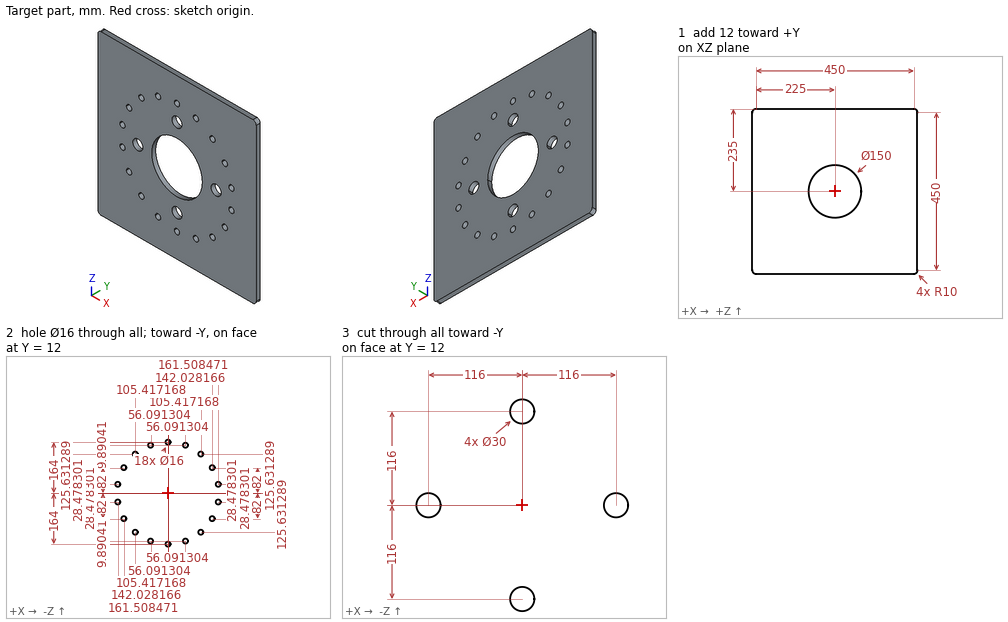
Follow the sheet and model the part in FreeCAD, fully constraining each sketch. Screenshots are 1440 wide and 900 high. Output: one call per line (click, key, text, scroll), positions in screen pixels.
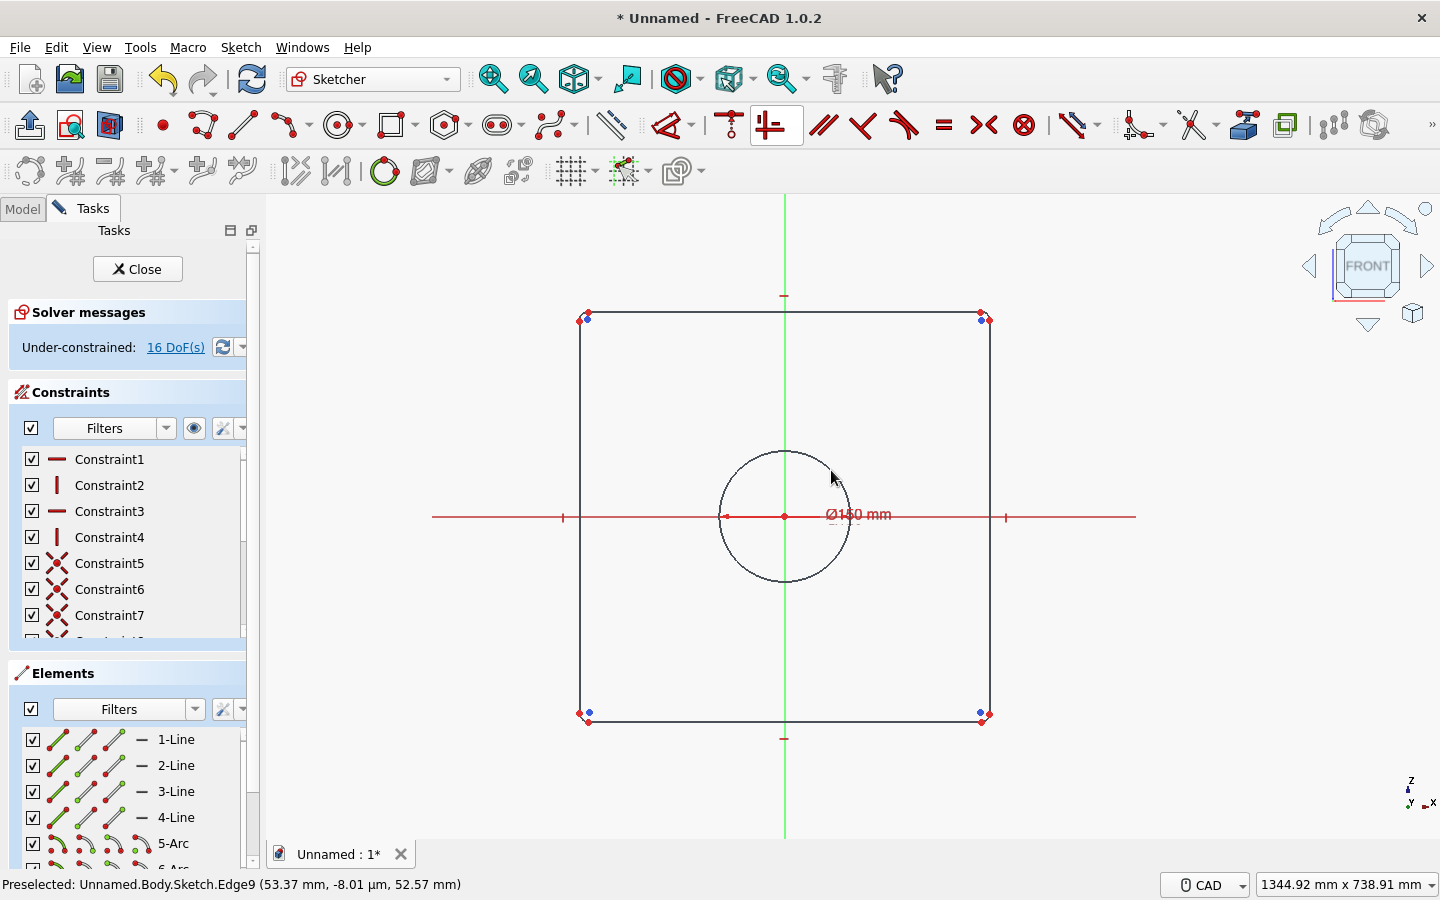
click(706, 312)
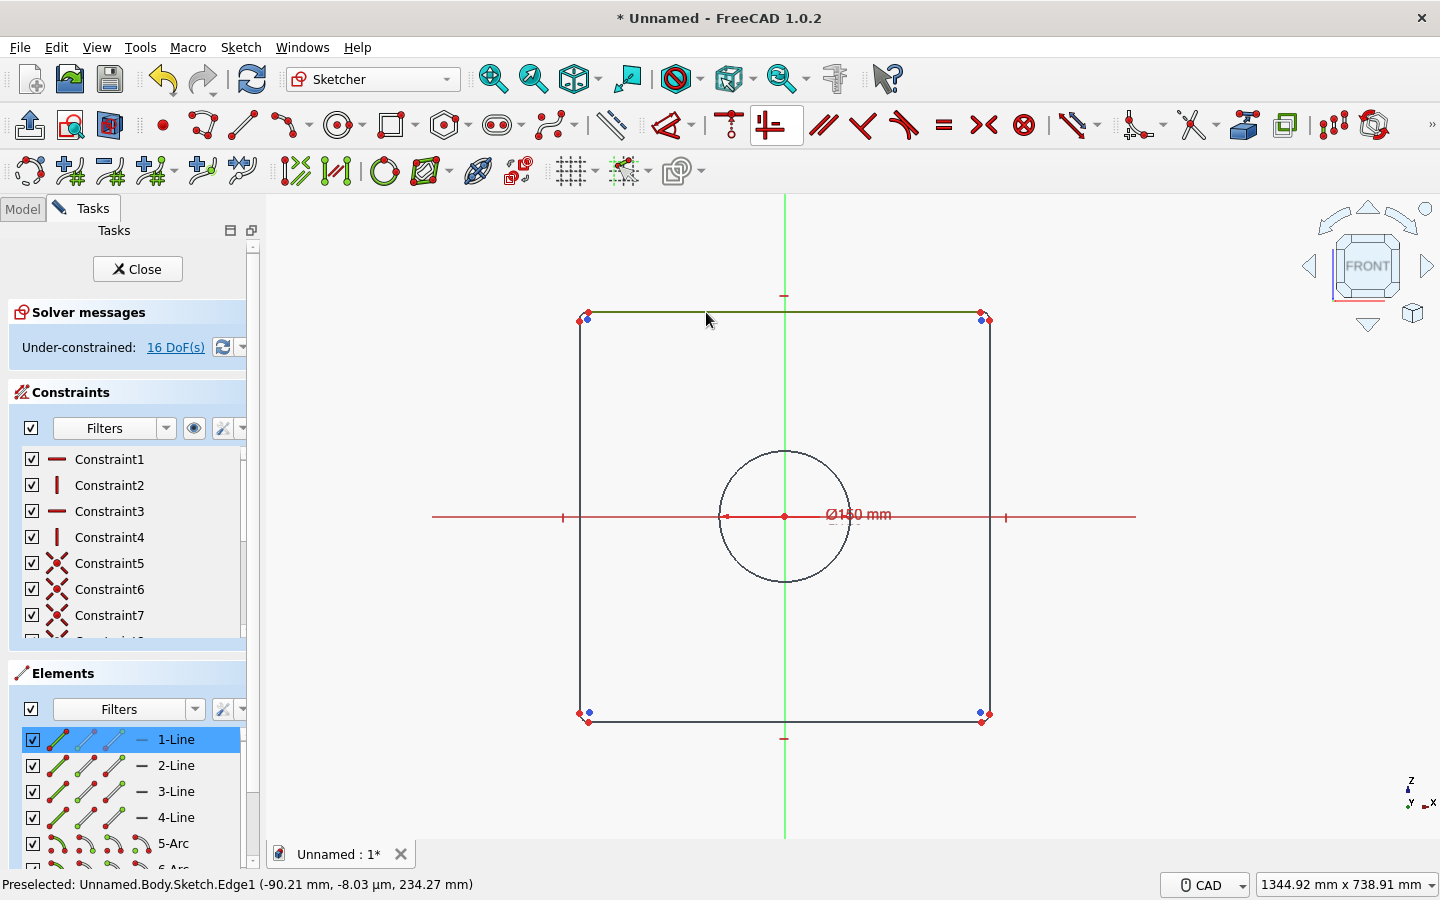
scroll(987, 314, up, 4)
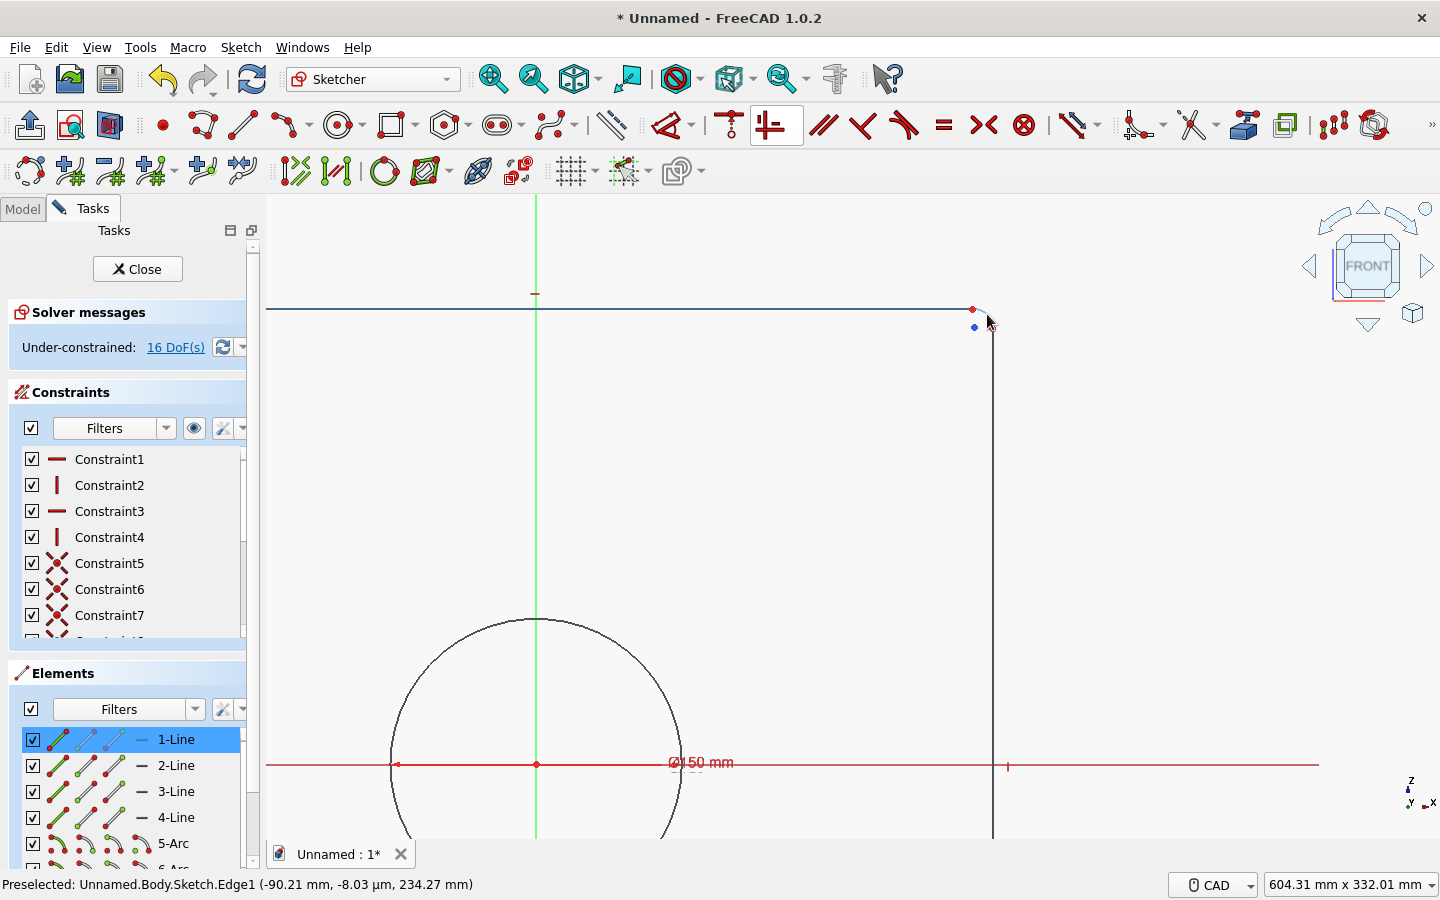
click(987, 314)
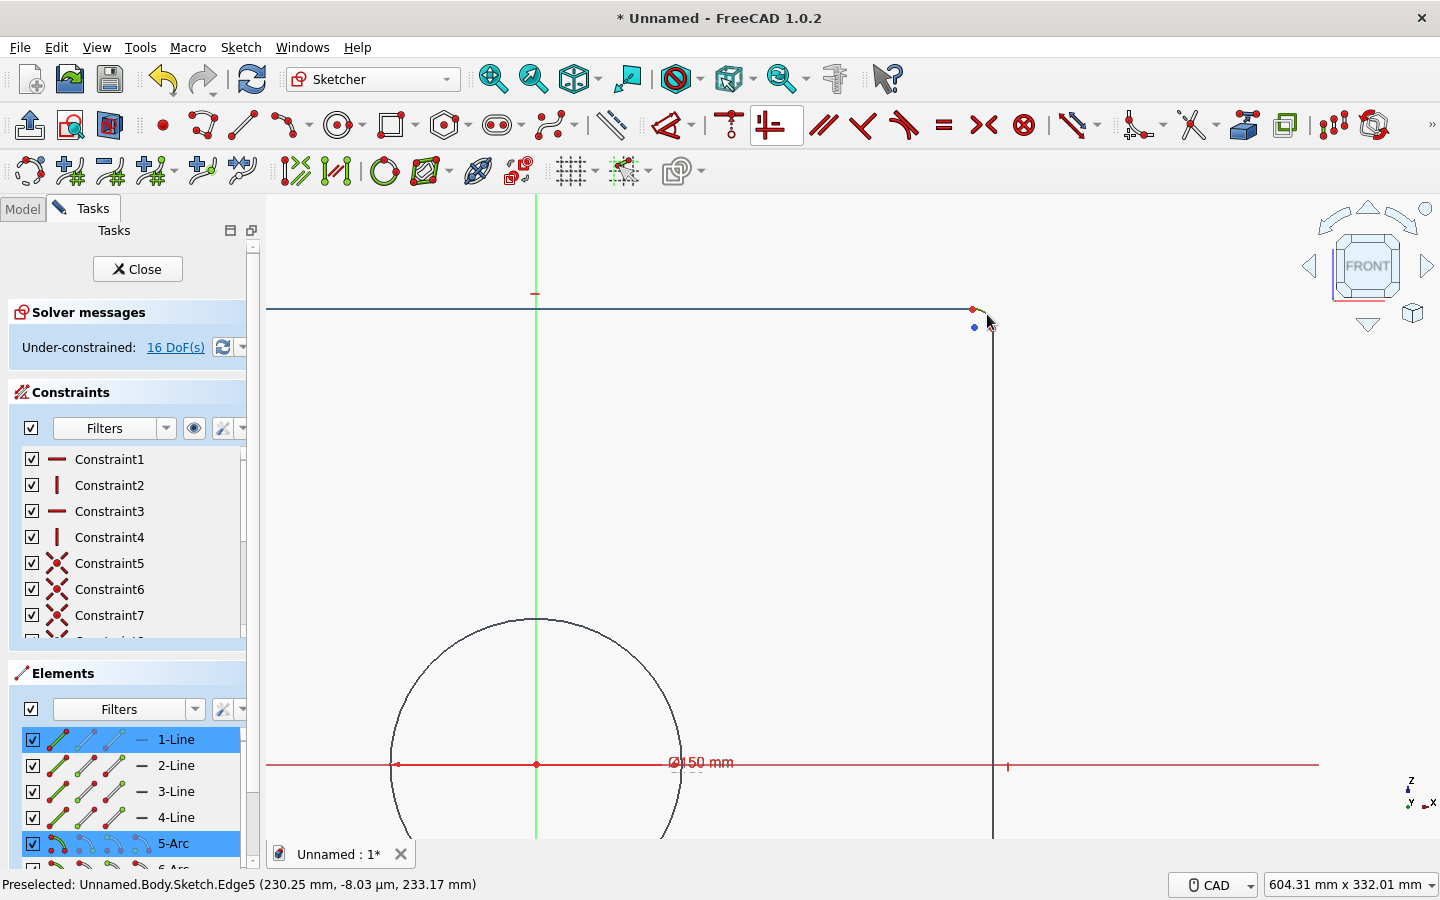
key(t)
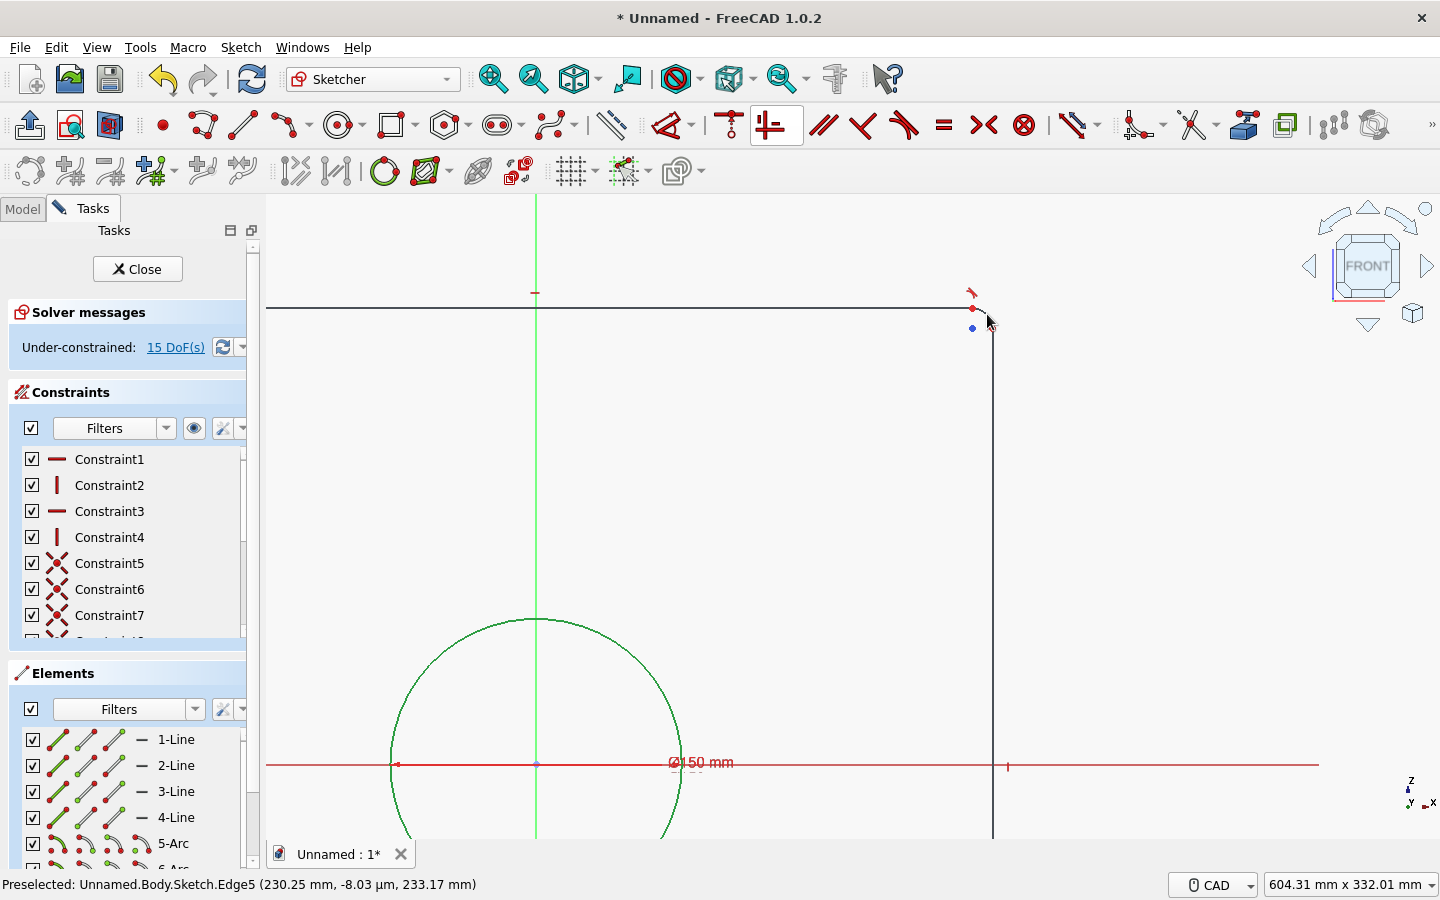
click(361, 308)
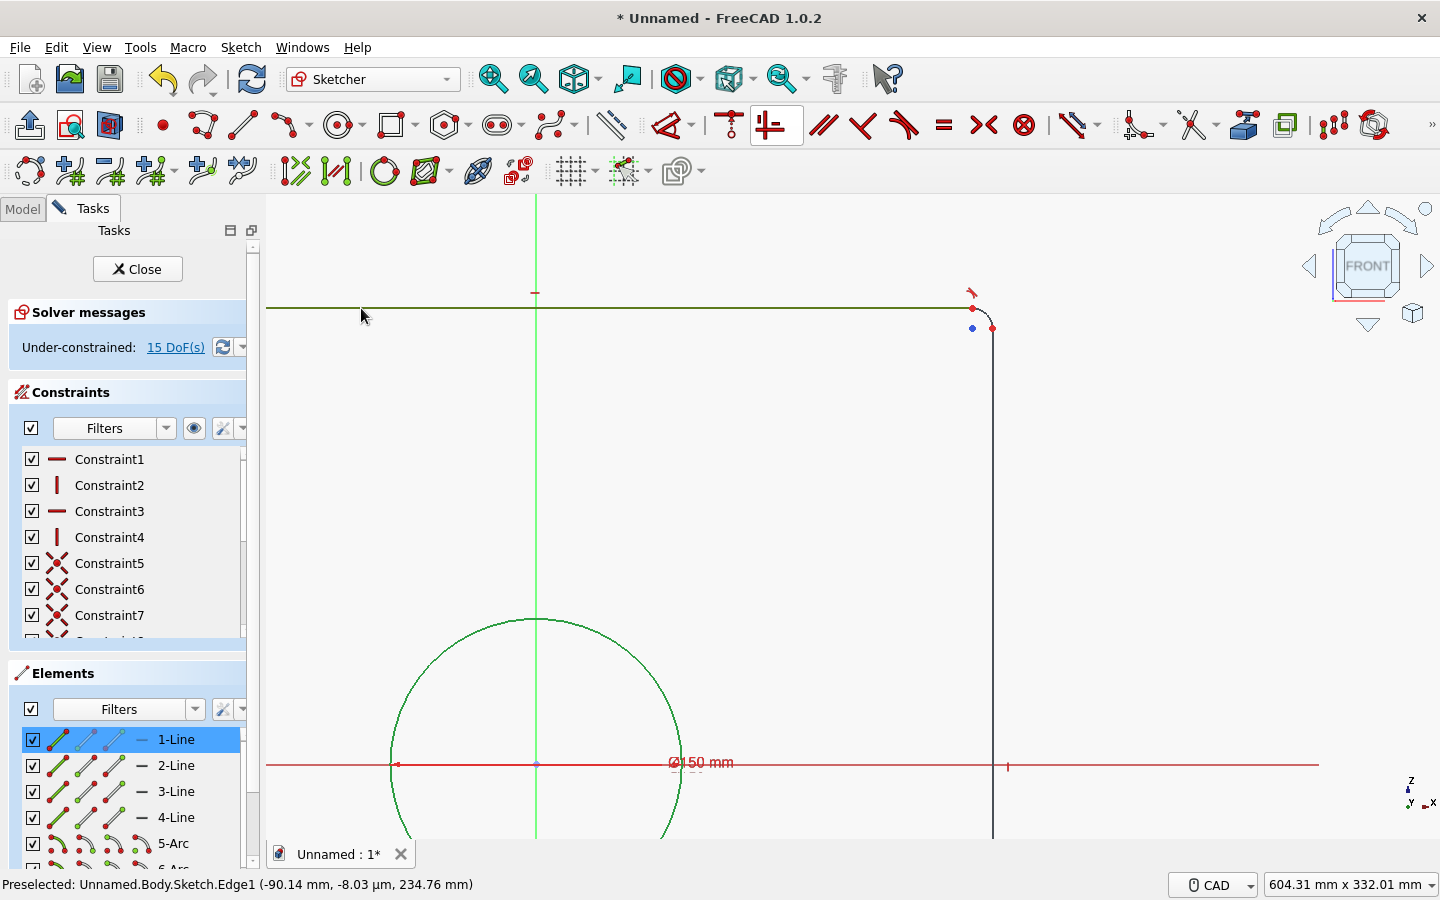
scroll(987, 314, down, 4)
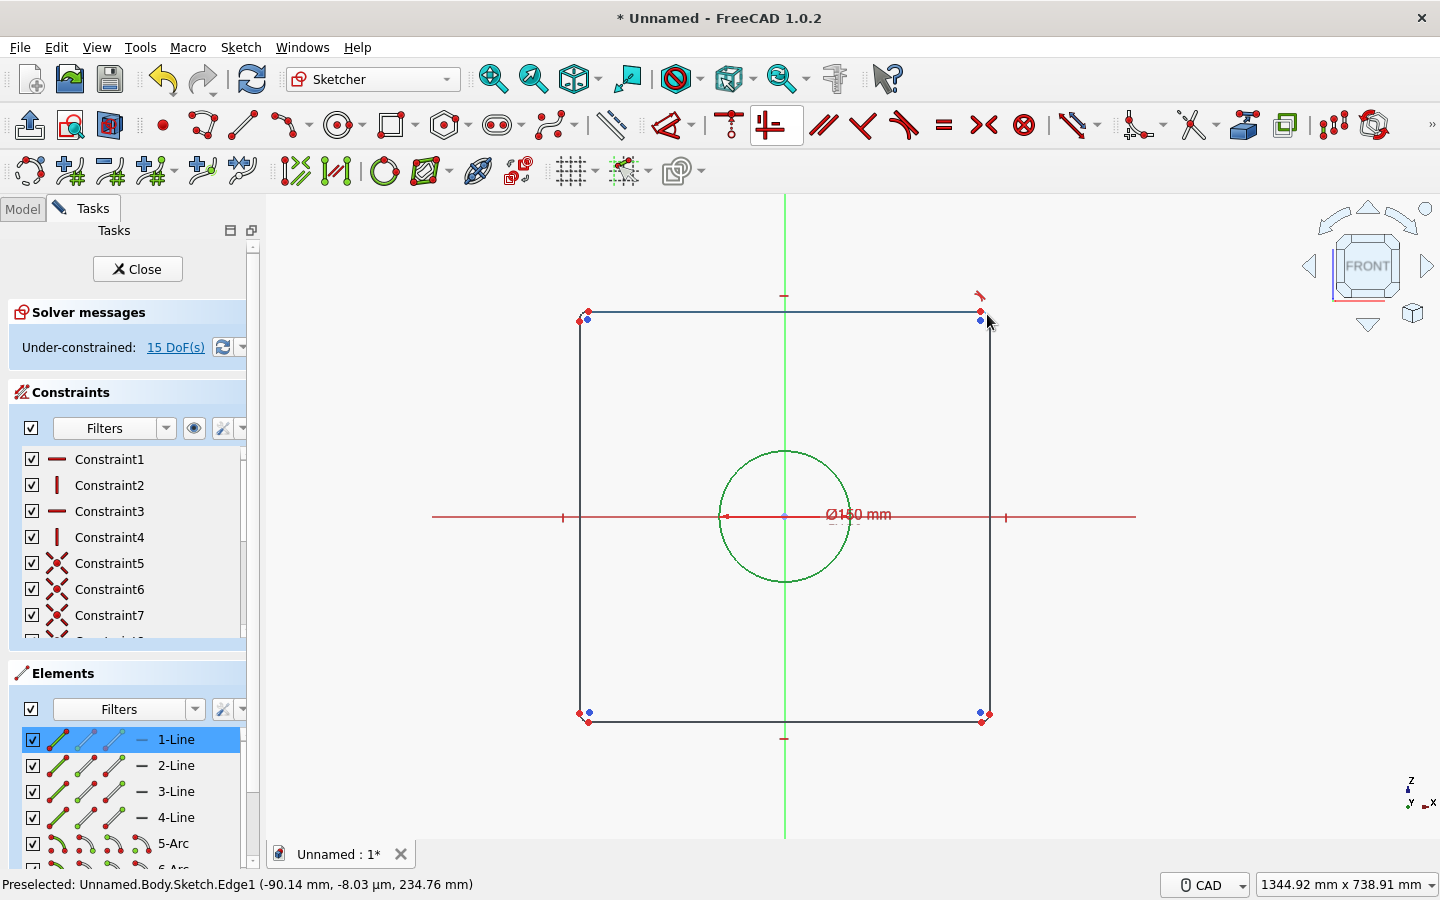
scroll(584, 312, up, 6)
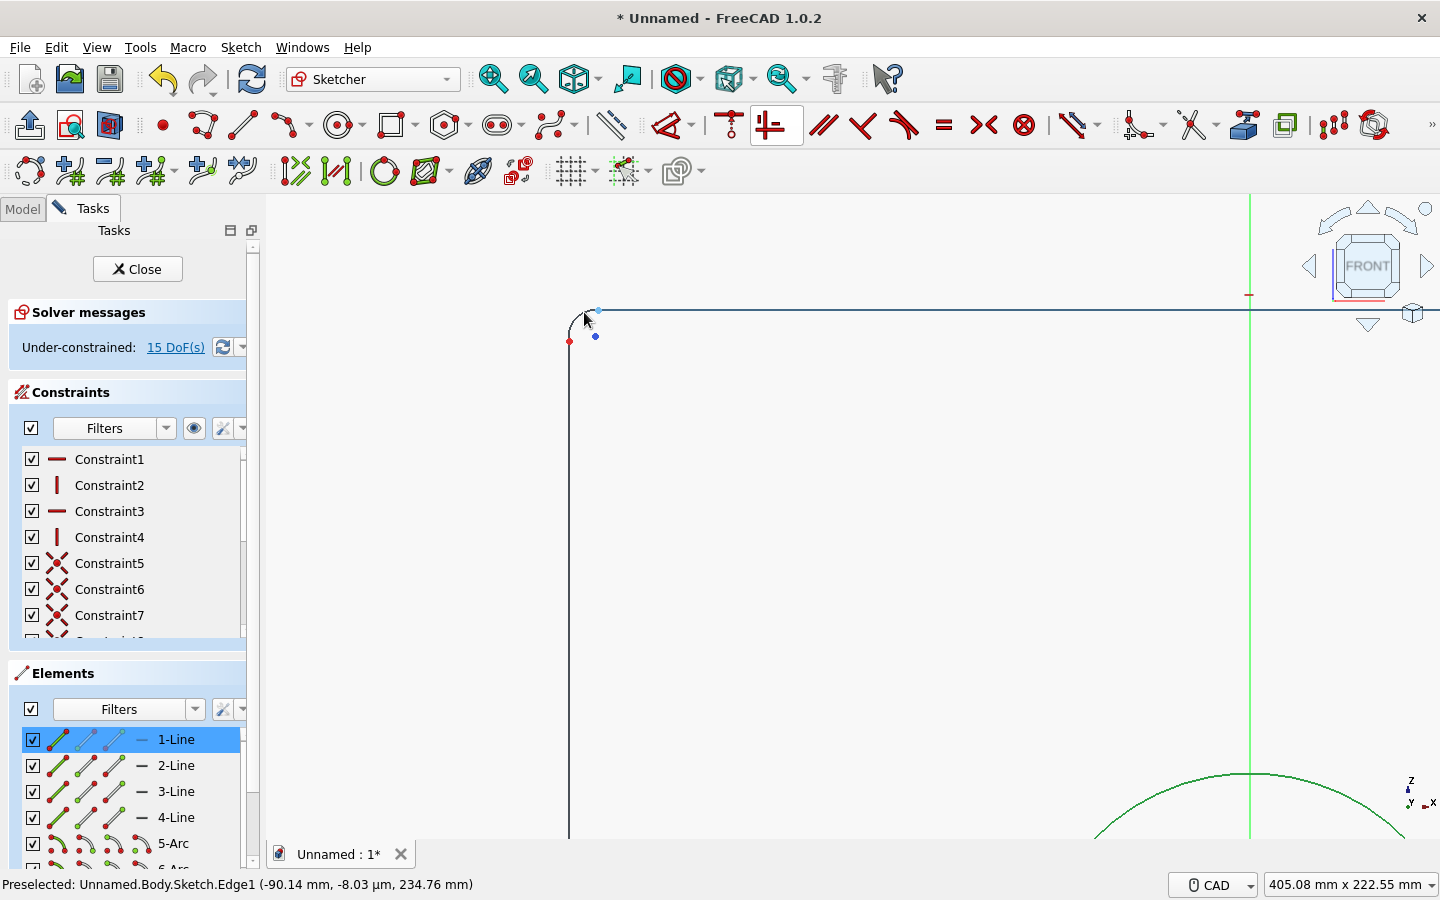
click(584, 313)